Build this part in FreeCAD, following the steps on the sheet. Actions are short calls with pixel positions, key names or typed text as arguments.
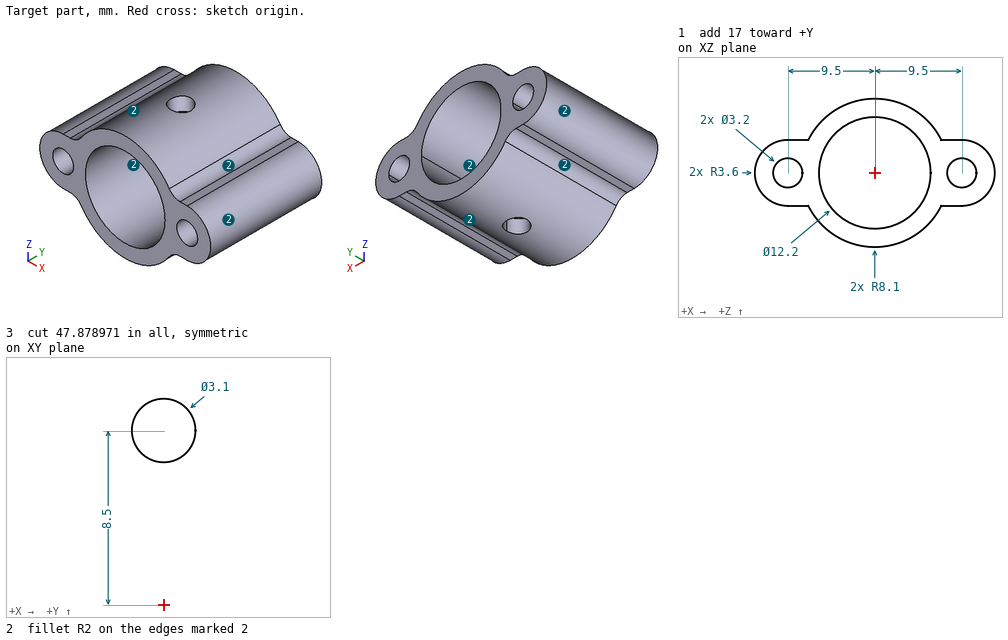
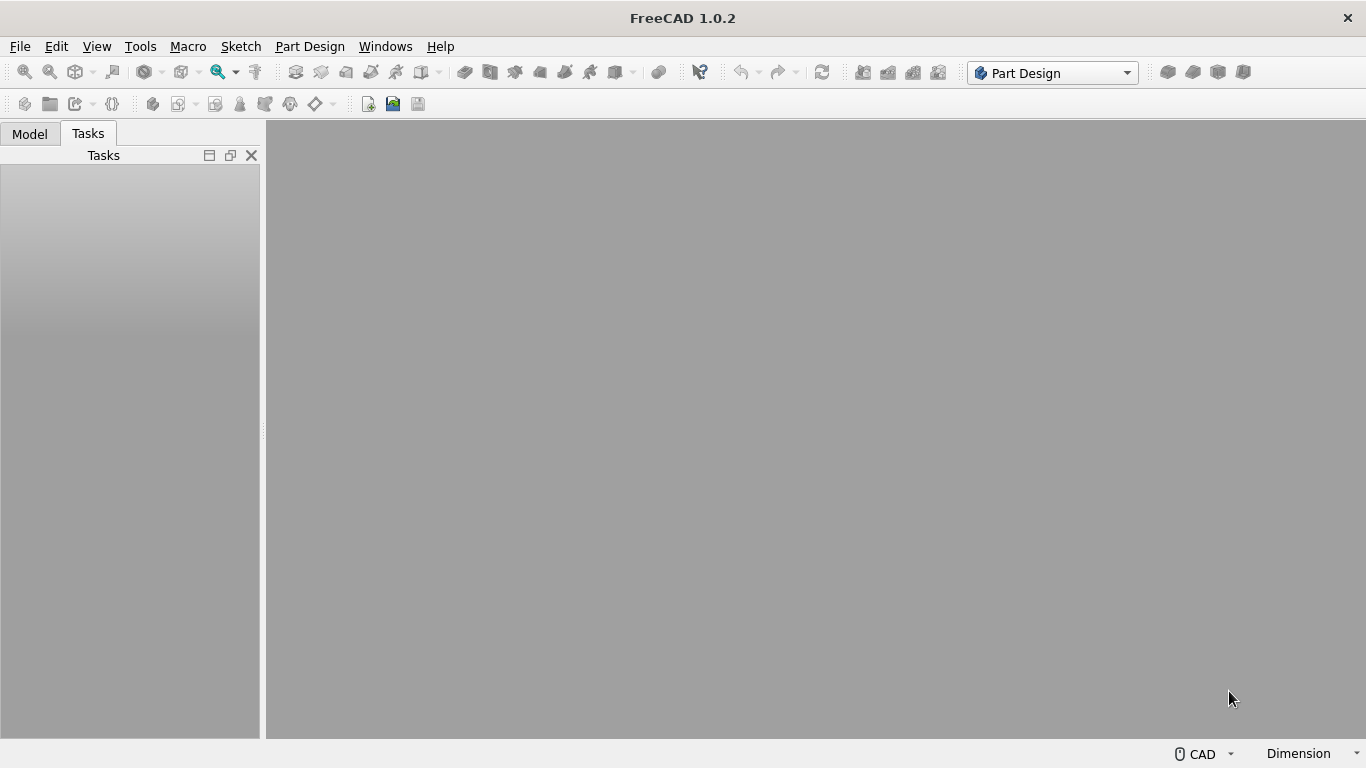
key(ctrl+n)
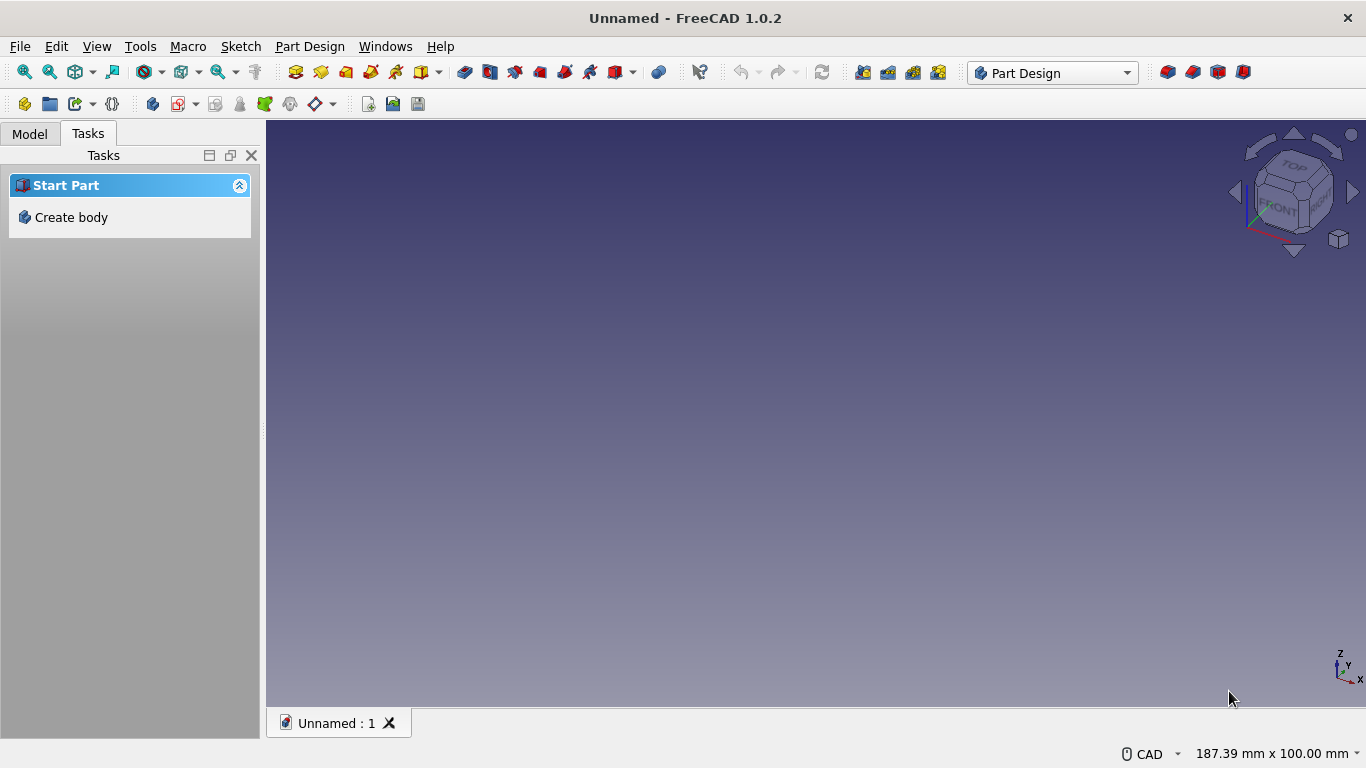
click(178, 104)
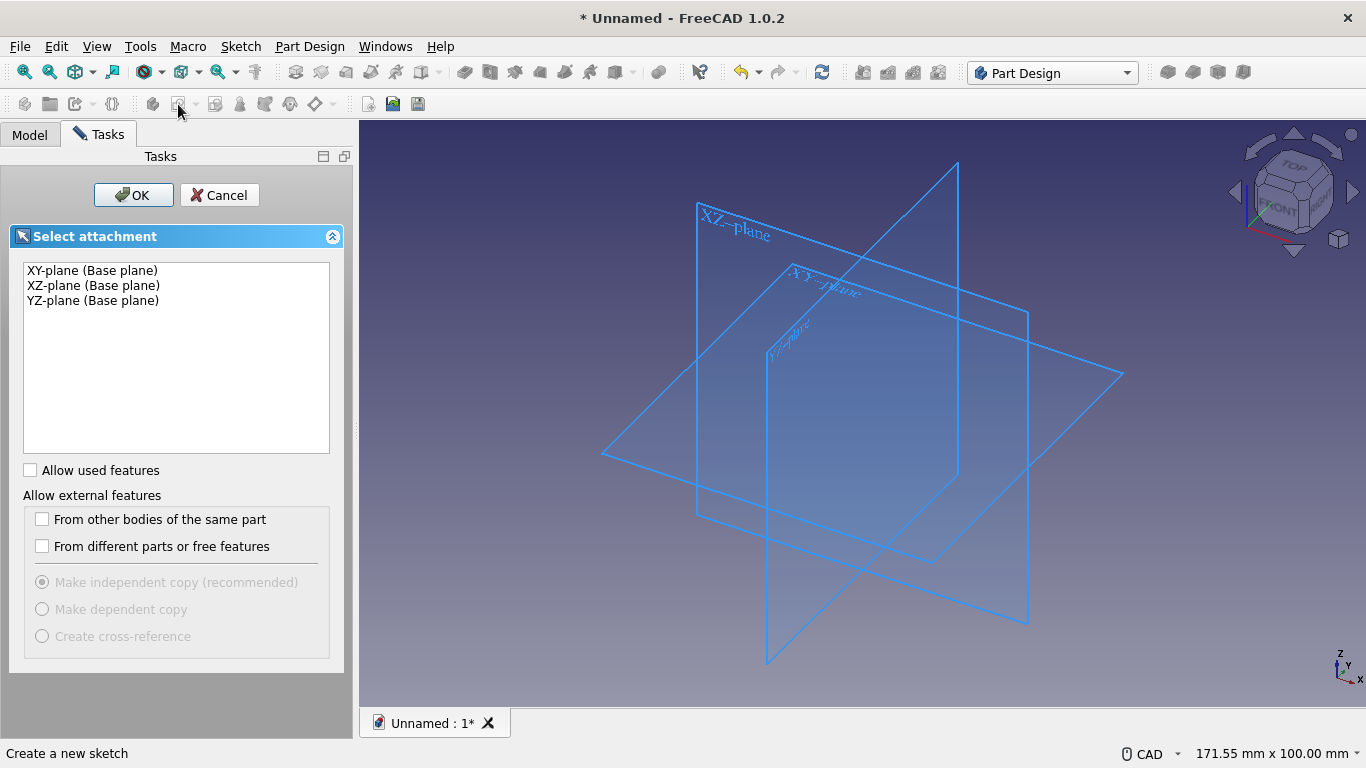
click(84, 286)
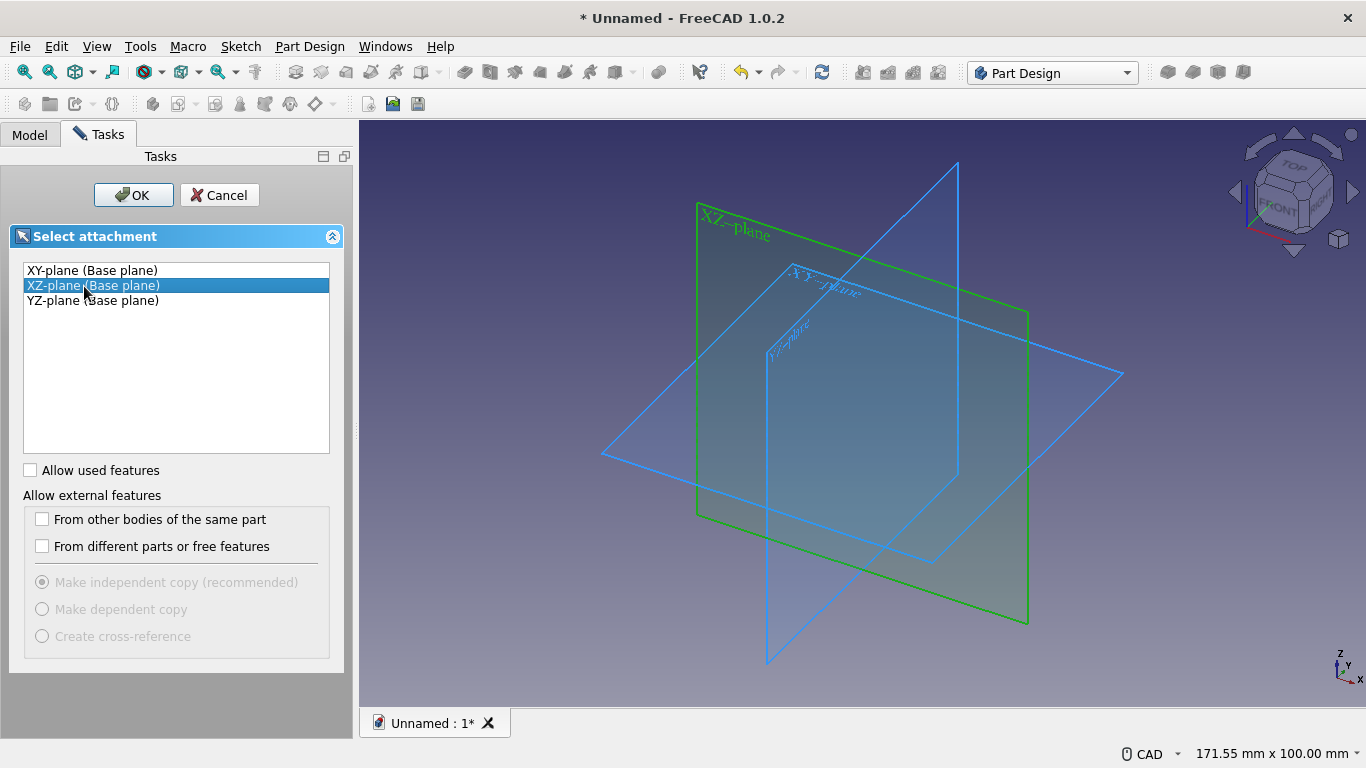
click(134, 195)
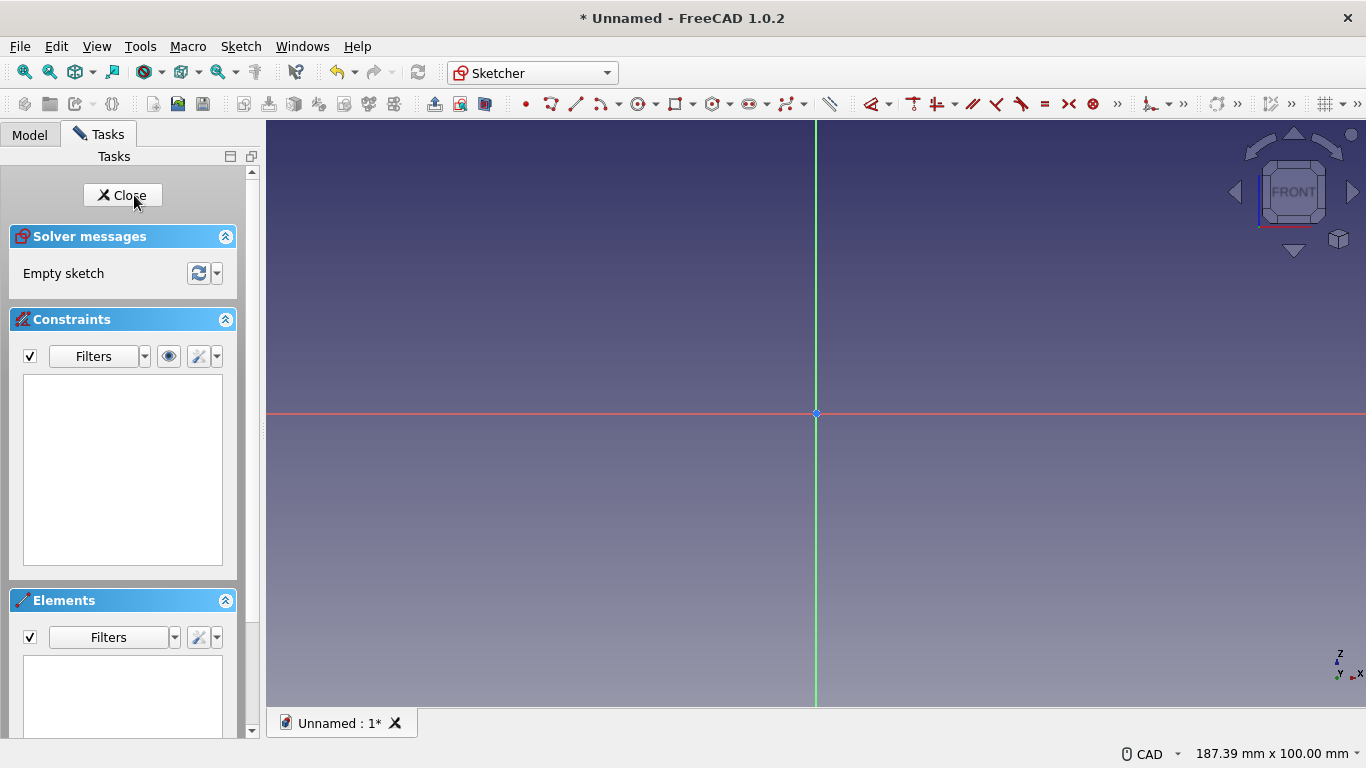
scroll(838, 414, up, 7)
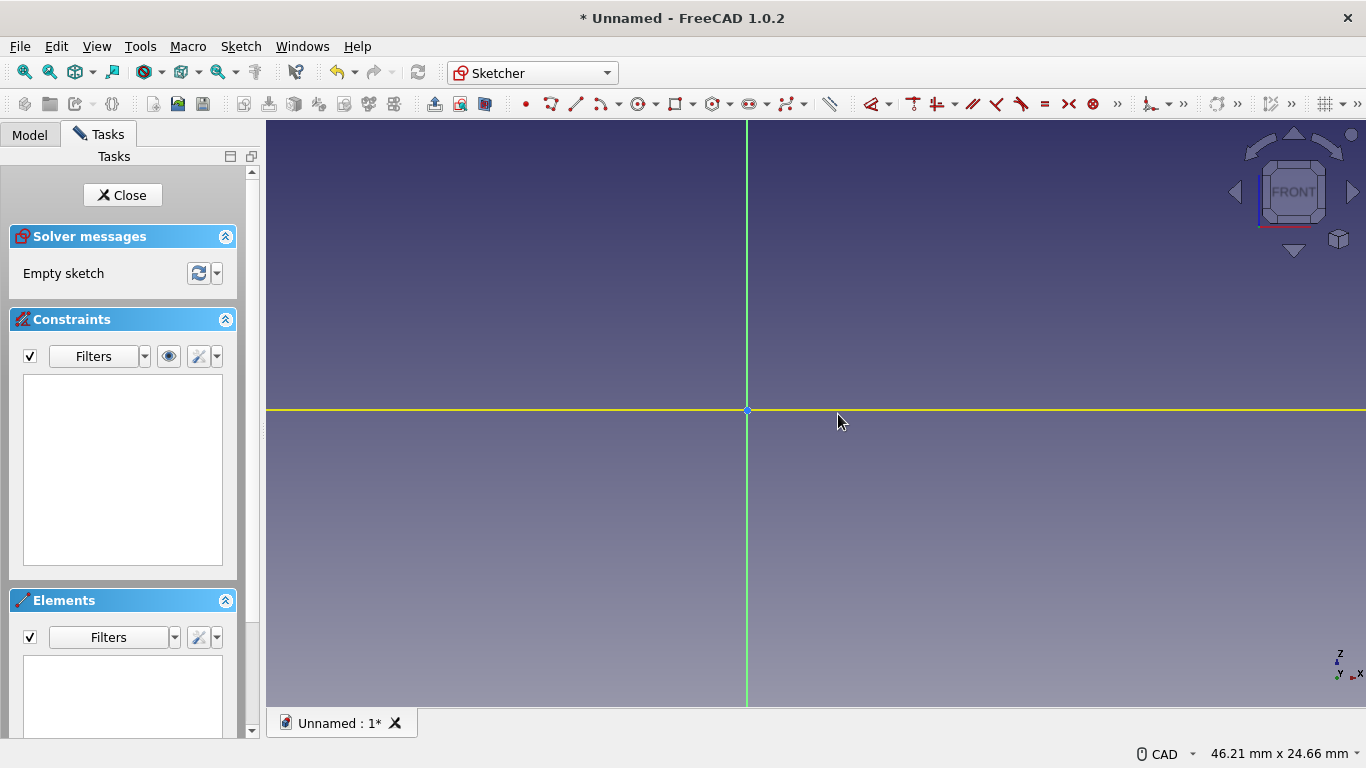
key(g)
key(l)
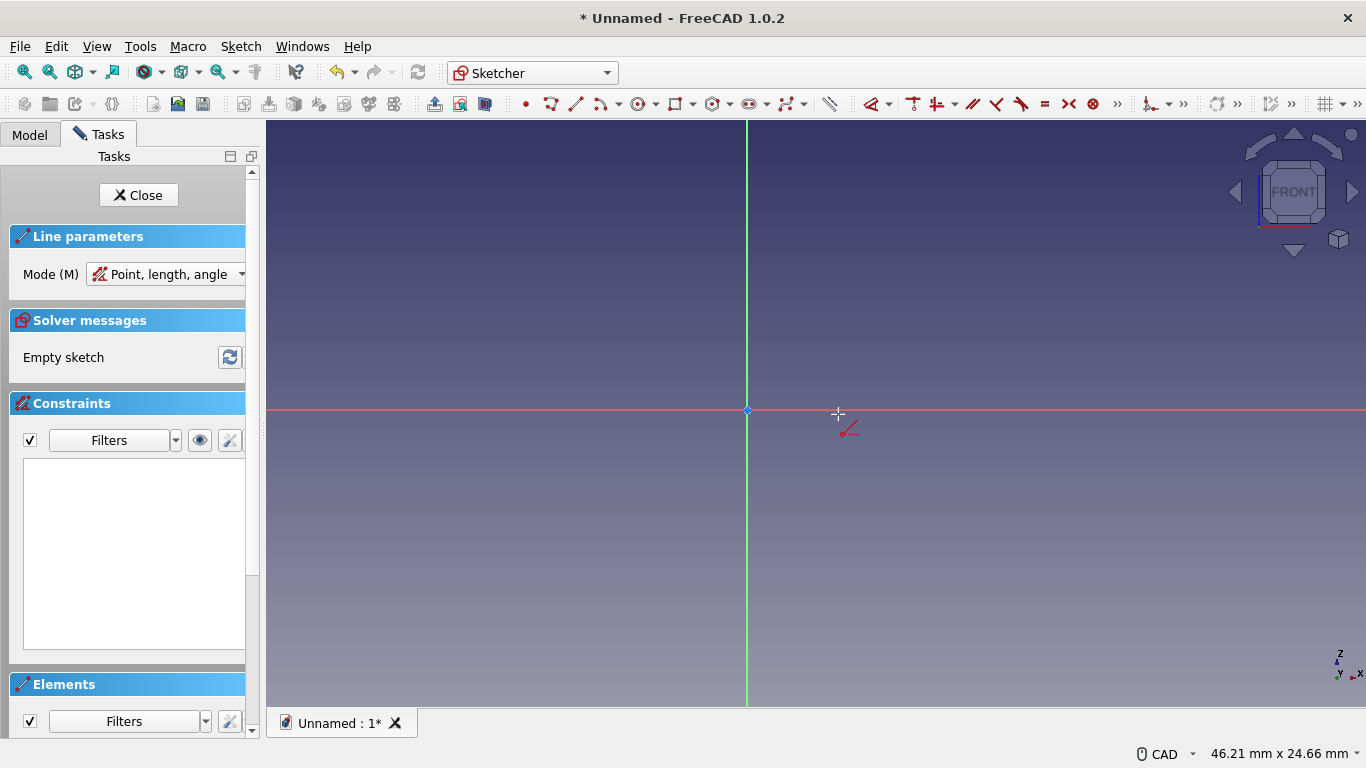
click(973, 496)
click(920, 496)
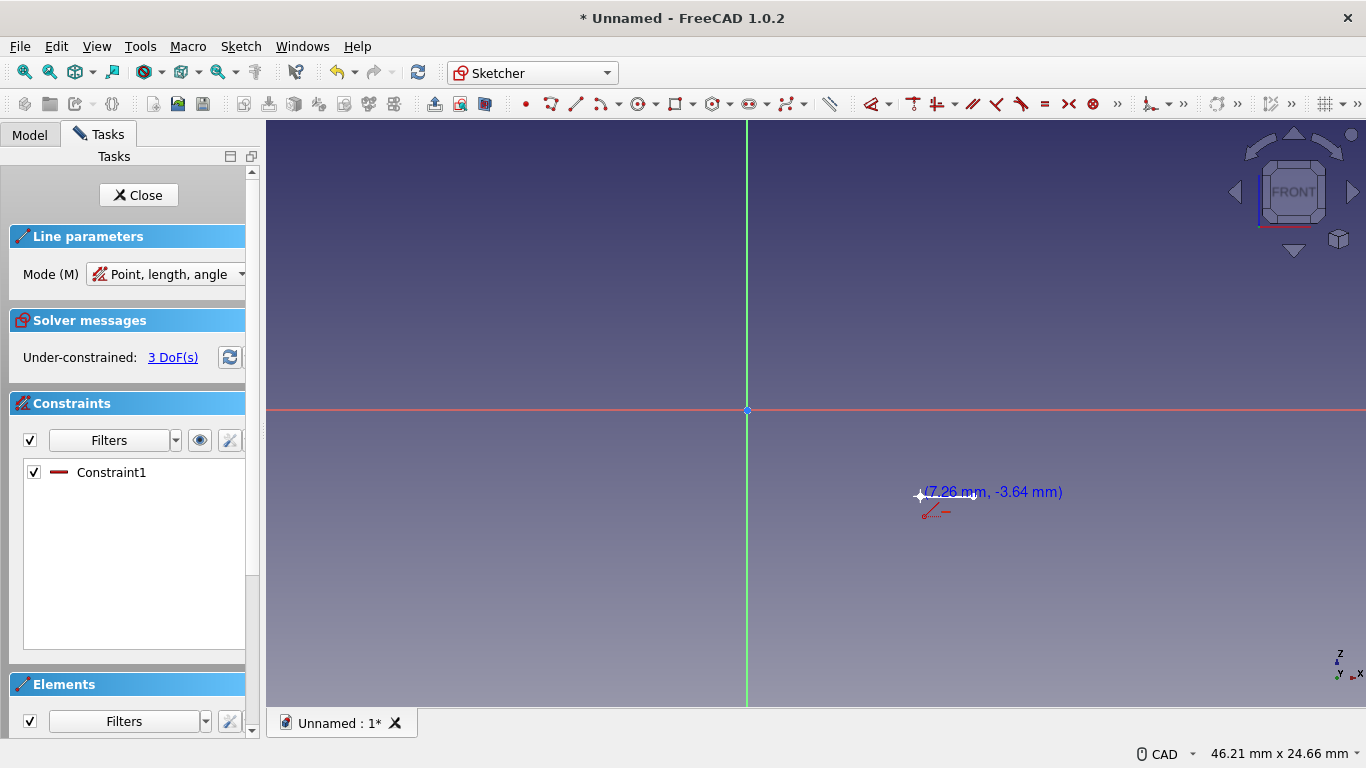
click(574, 496)
click(521, 496)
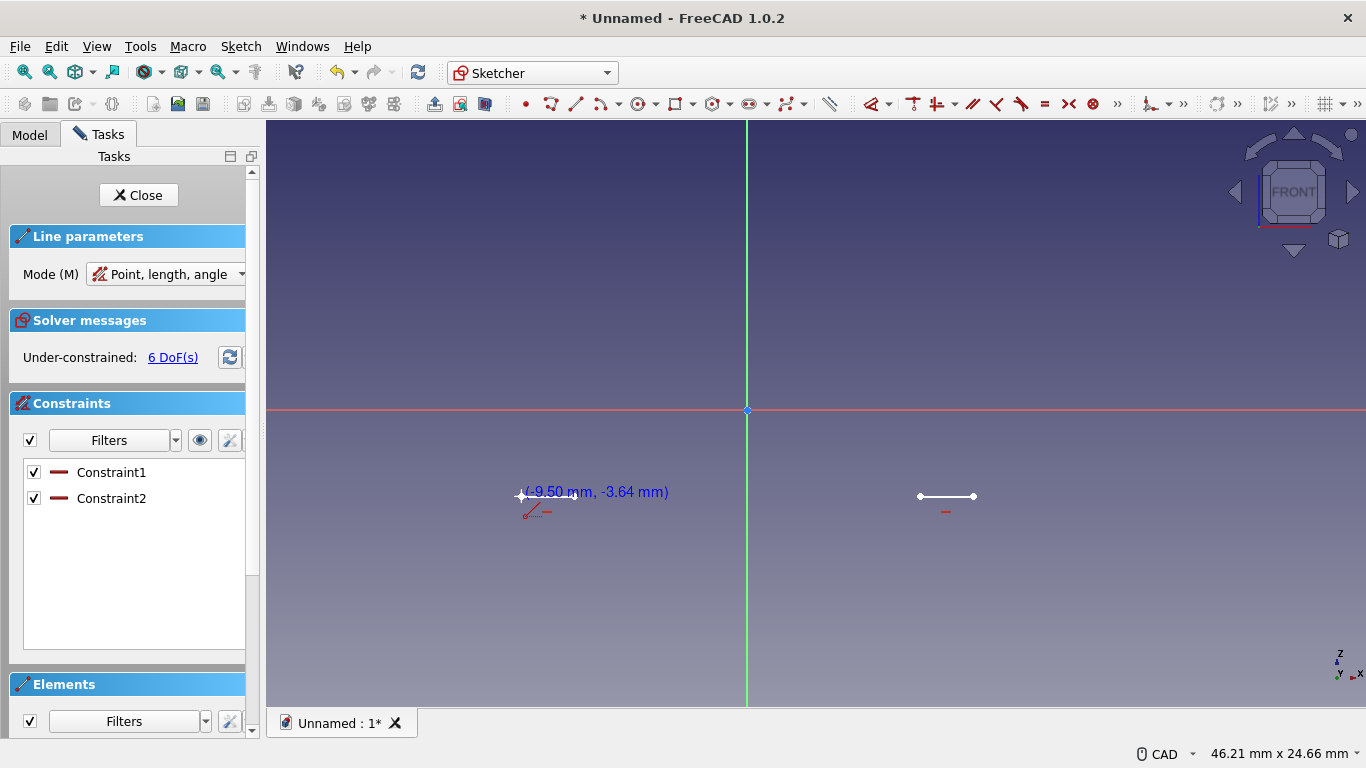
click(521, 325)
click(574, 325)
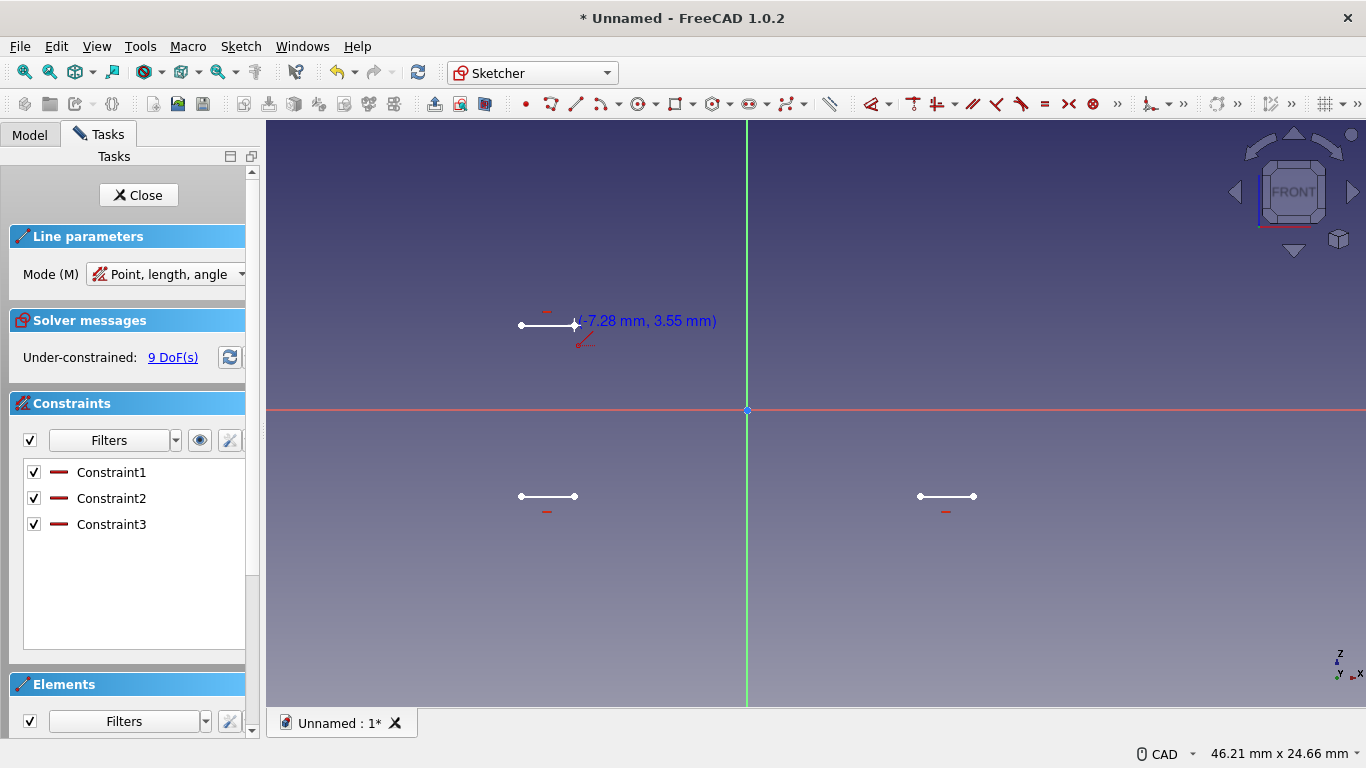
click(920, 325)
click(973, 325)